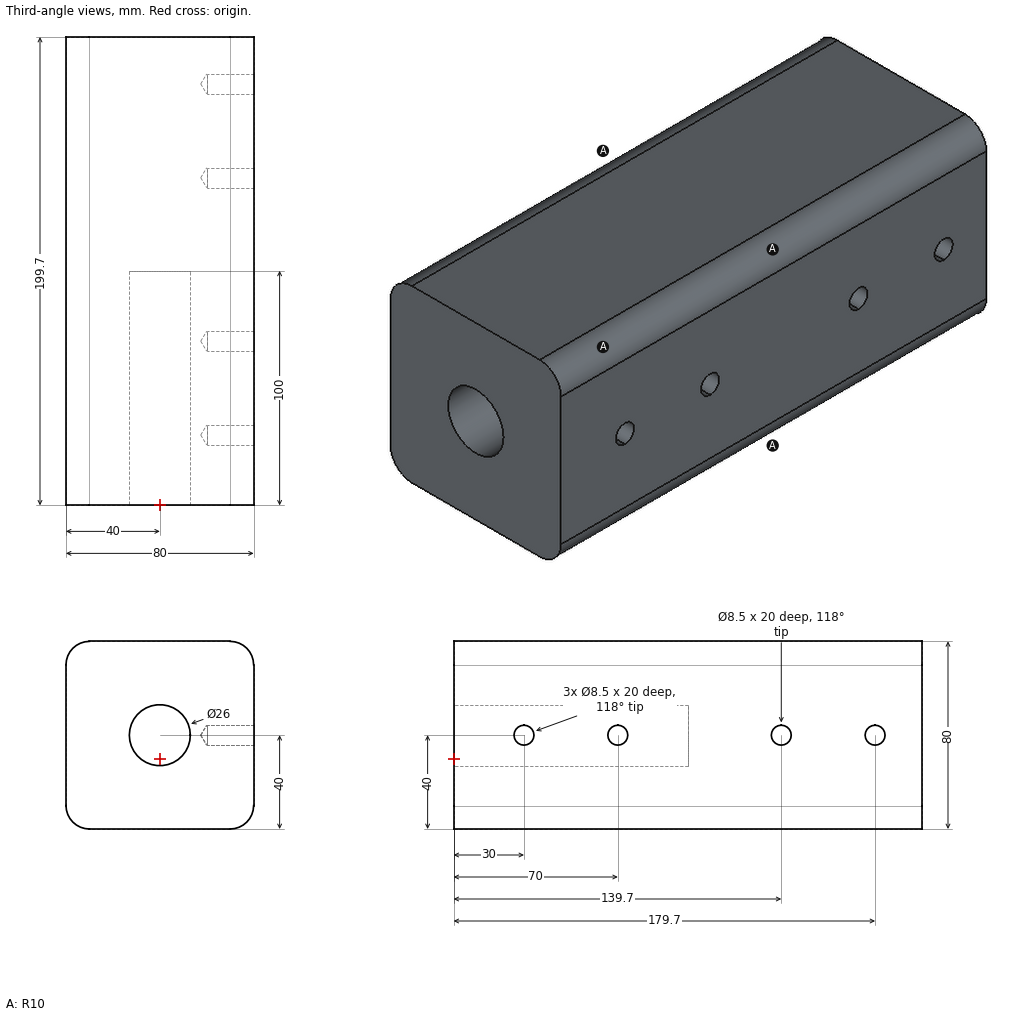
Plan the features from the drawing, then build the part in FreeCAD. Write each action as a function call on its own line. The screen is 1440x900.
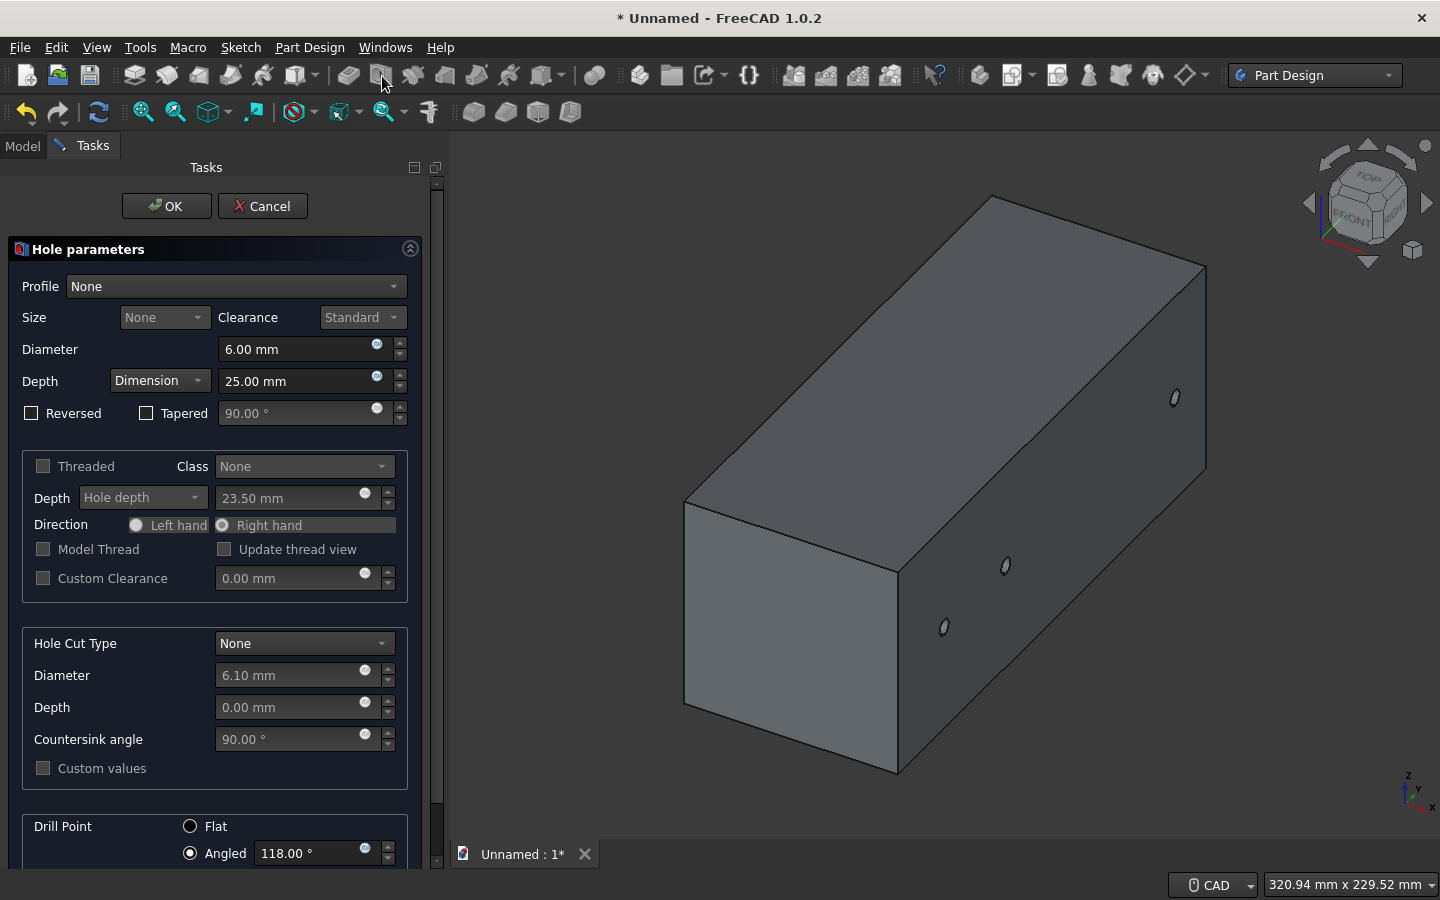
triple_click(305, 349)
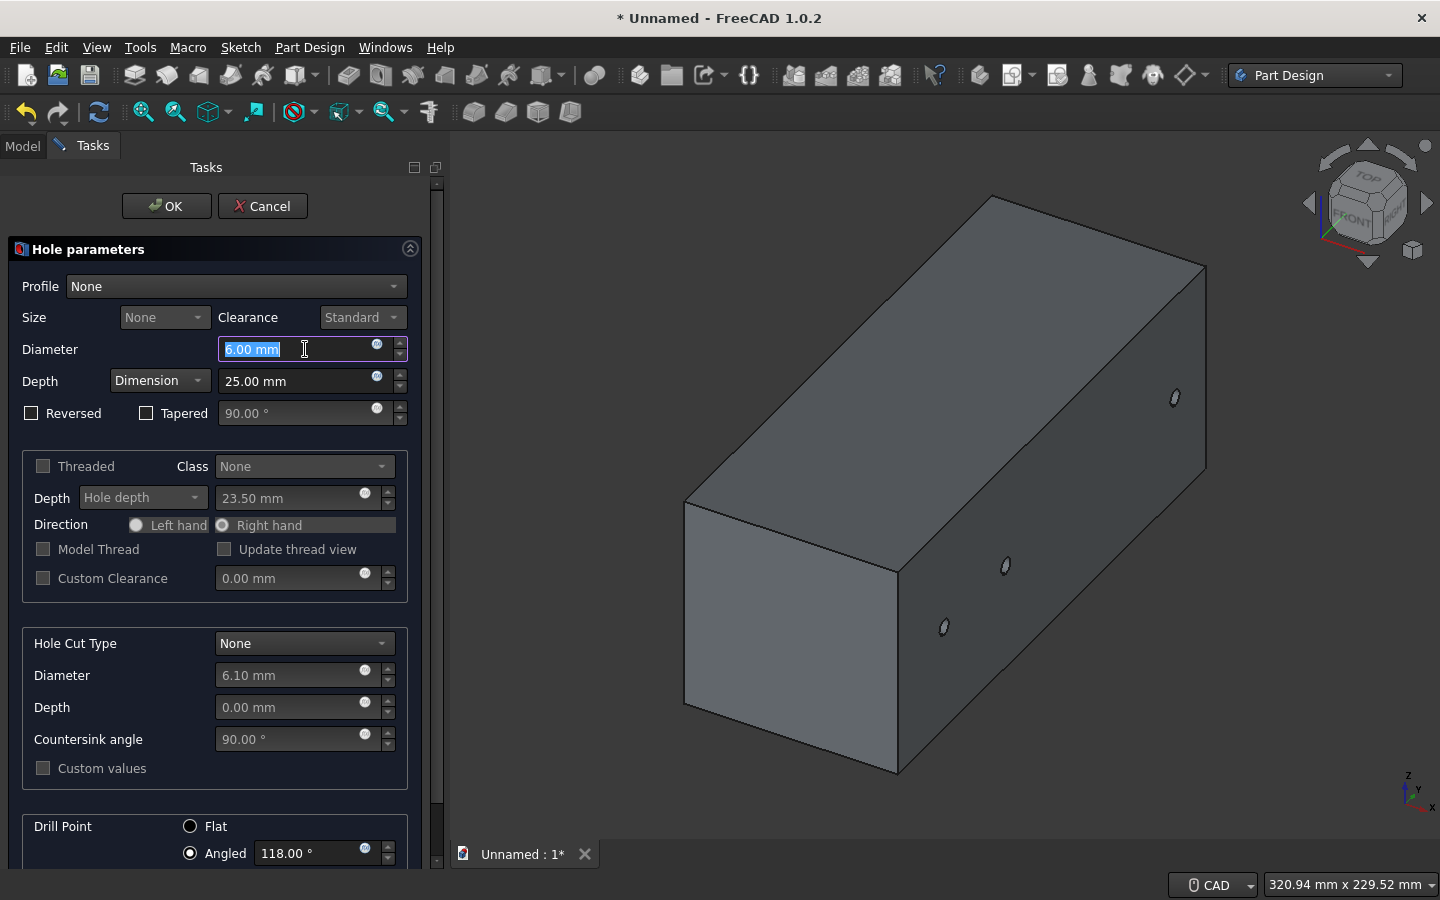
text(8.5)
key(Tab)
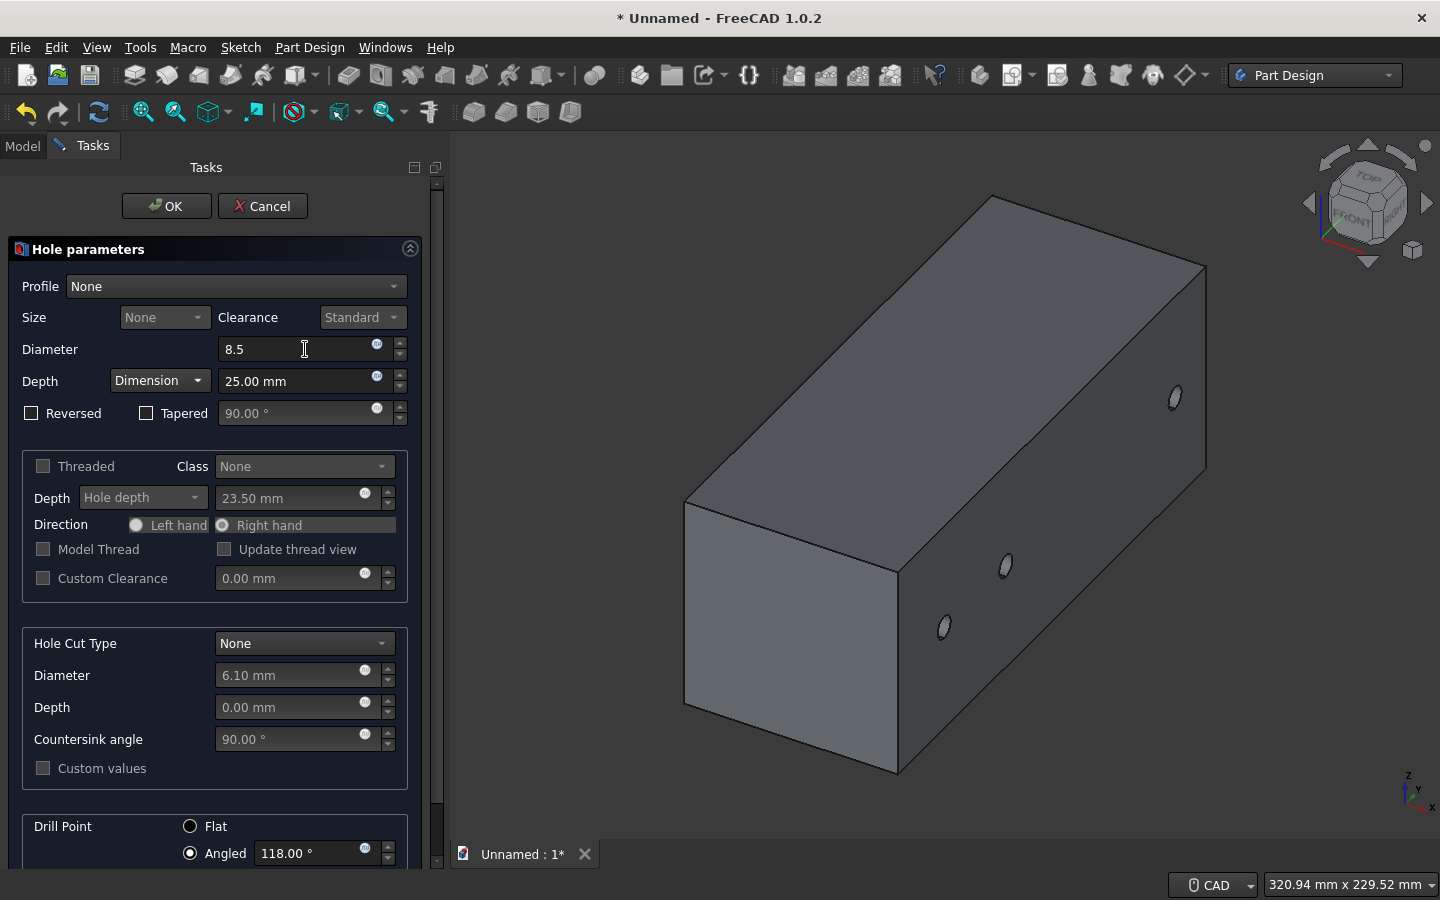
triple_click(305, 381)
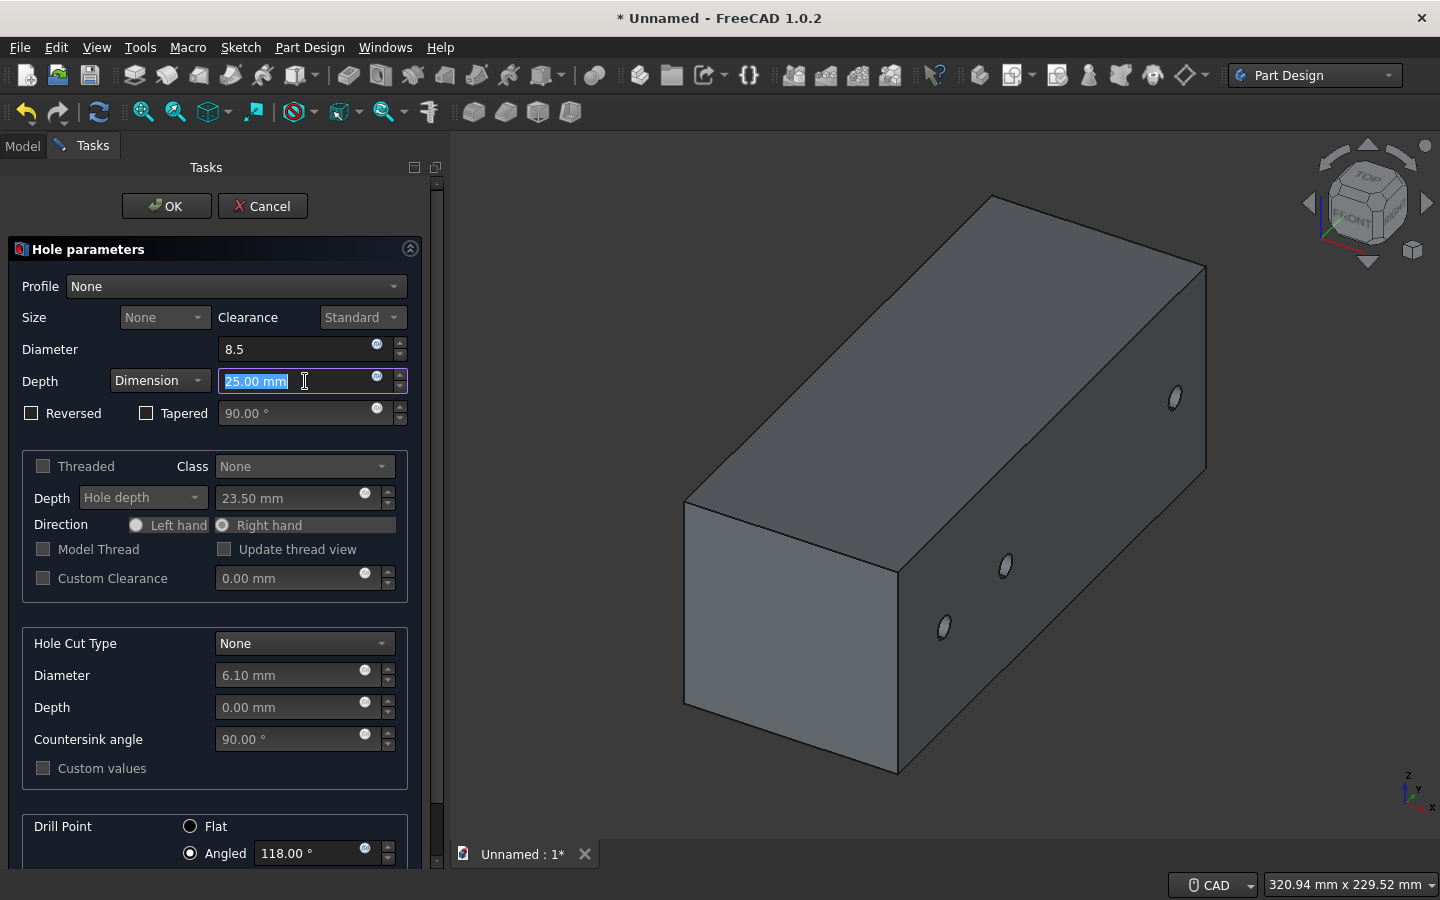
text(20)
key(Tab)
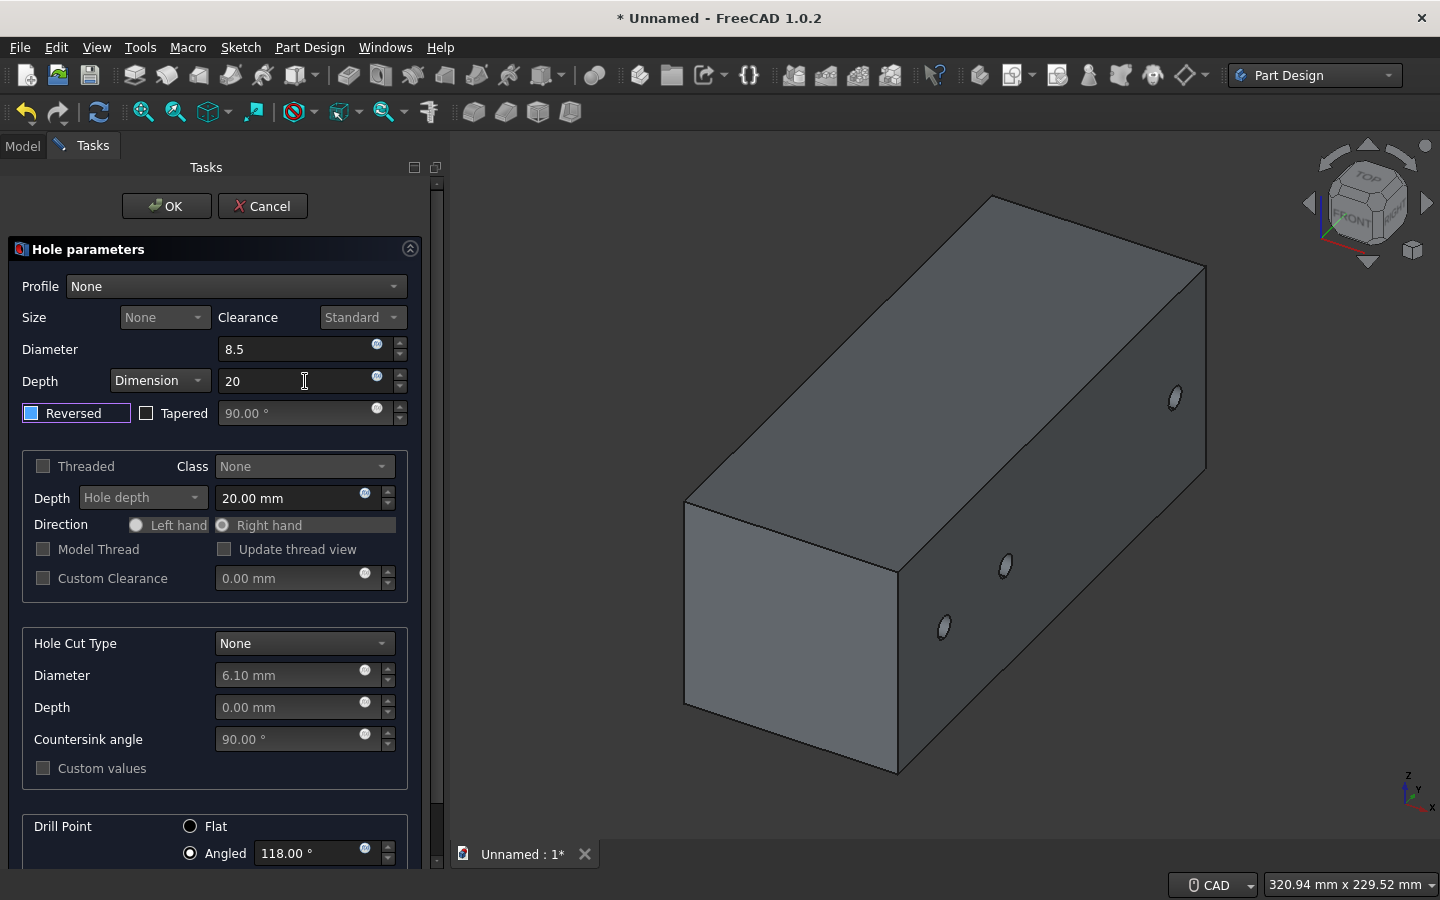
click(167, 206)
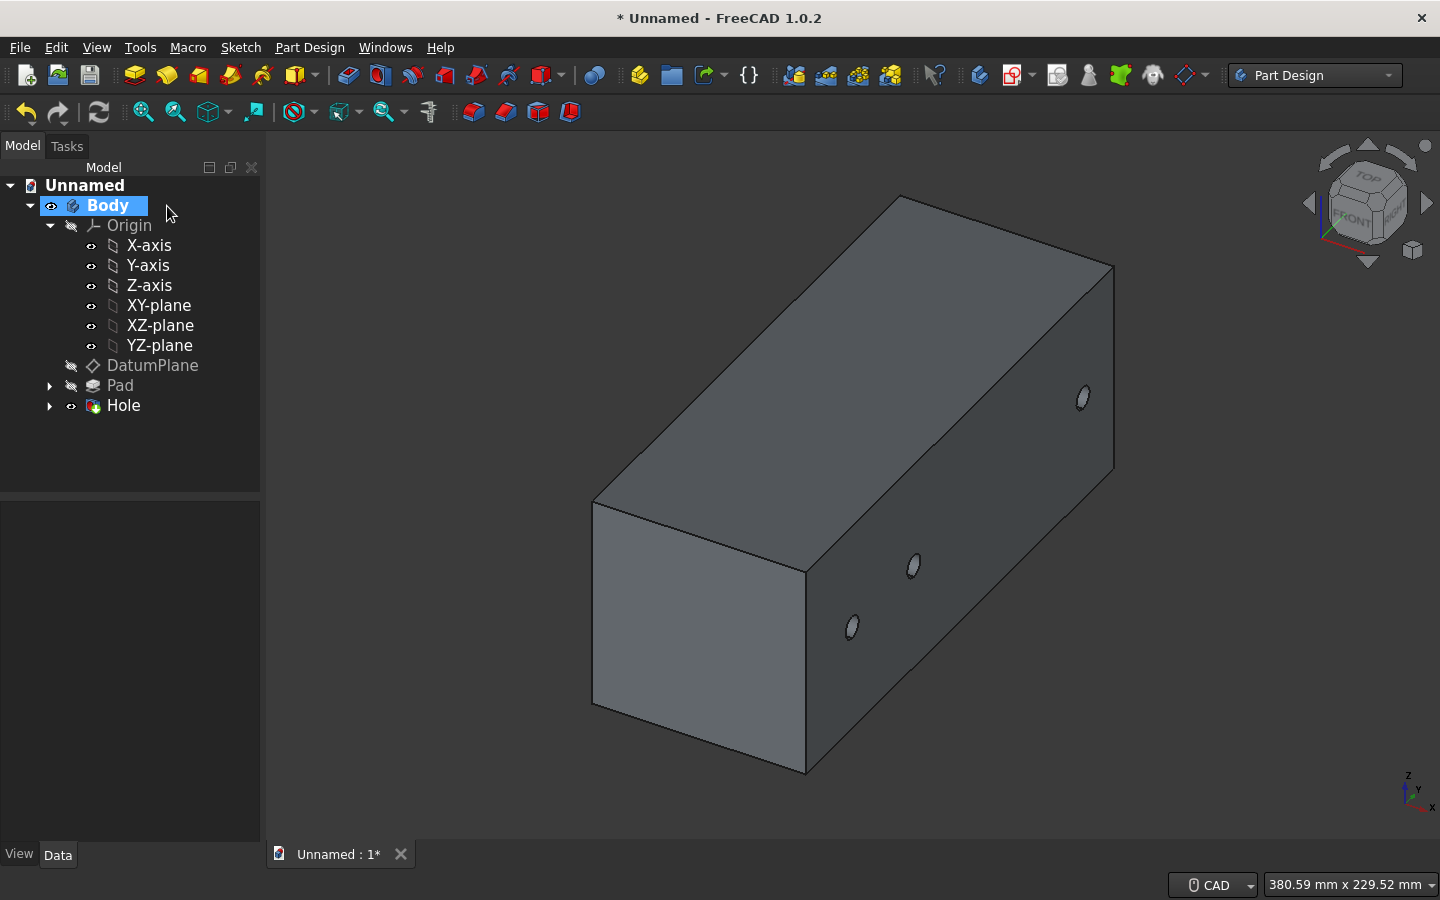
click(960, 418)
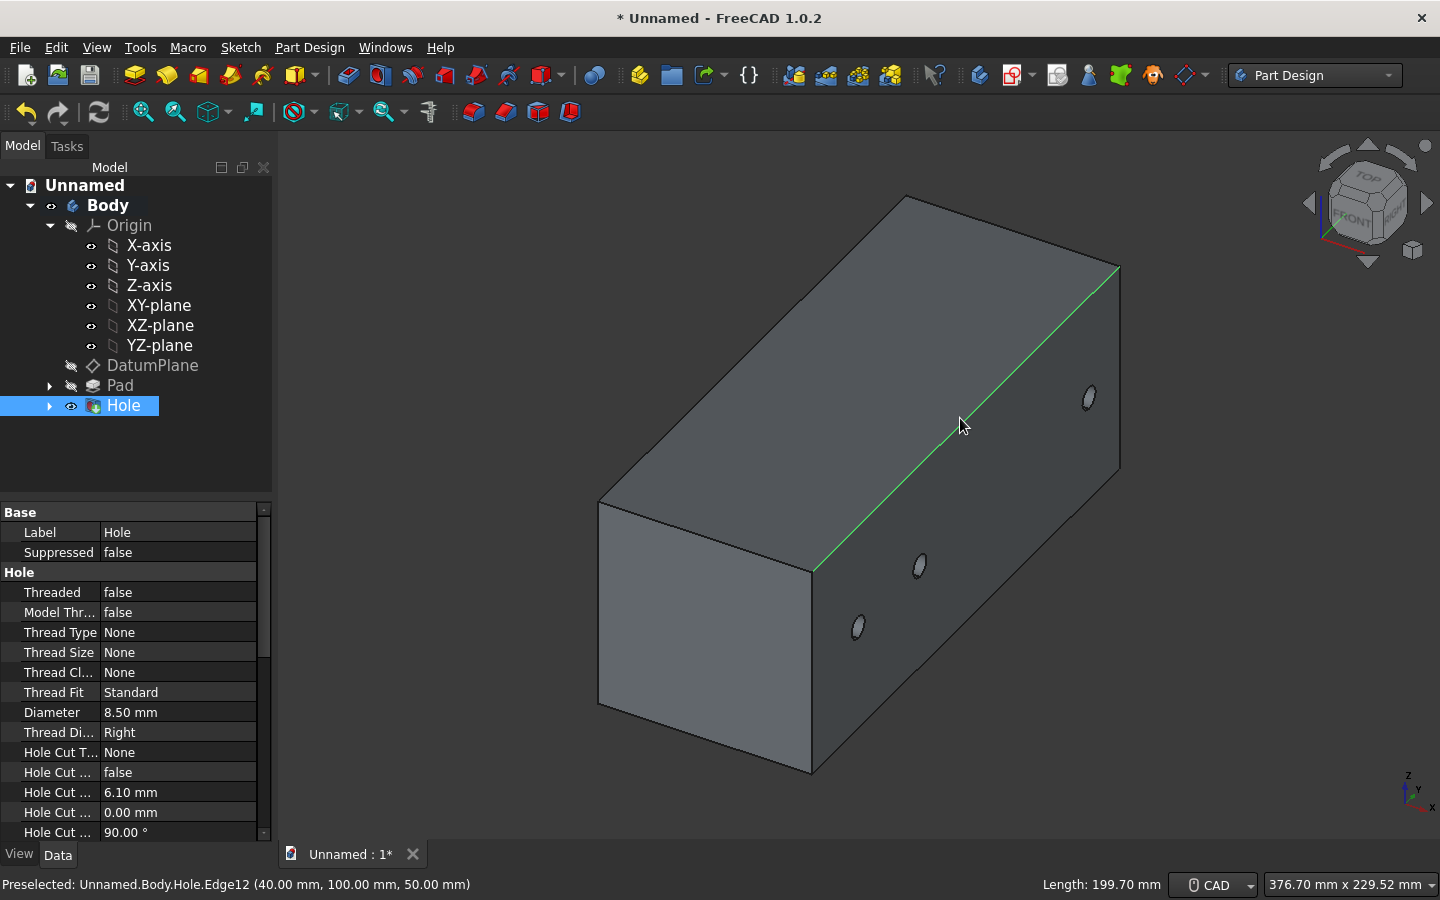
key(0)